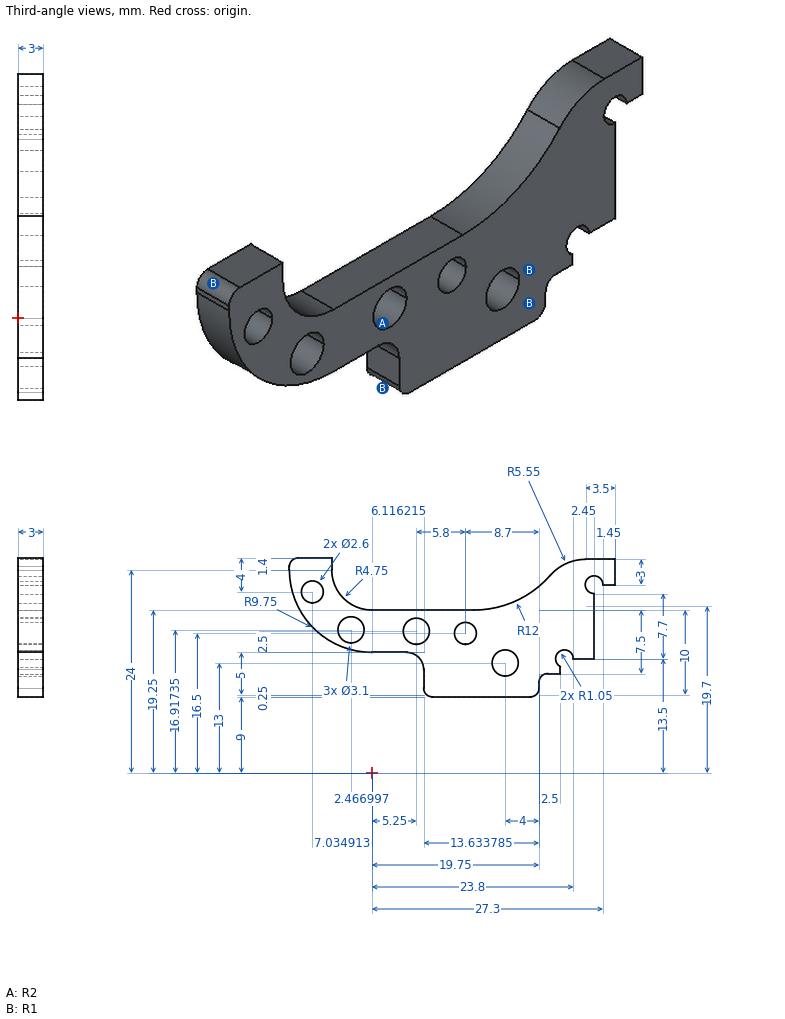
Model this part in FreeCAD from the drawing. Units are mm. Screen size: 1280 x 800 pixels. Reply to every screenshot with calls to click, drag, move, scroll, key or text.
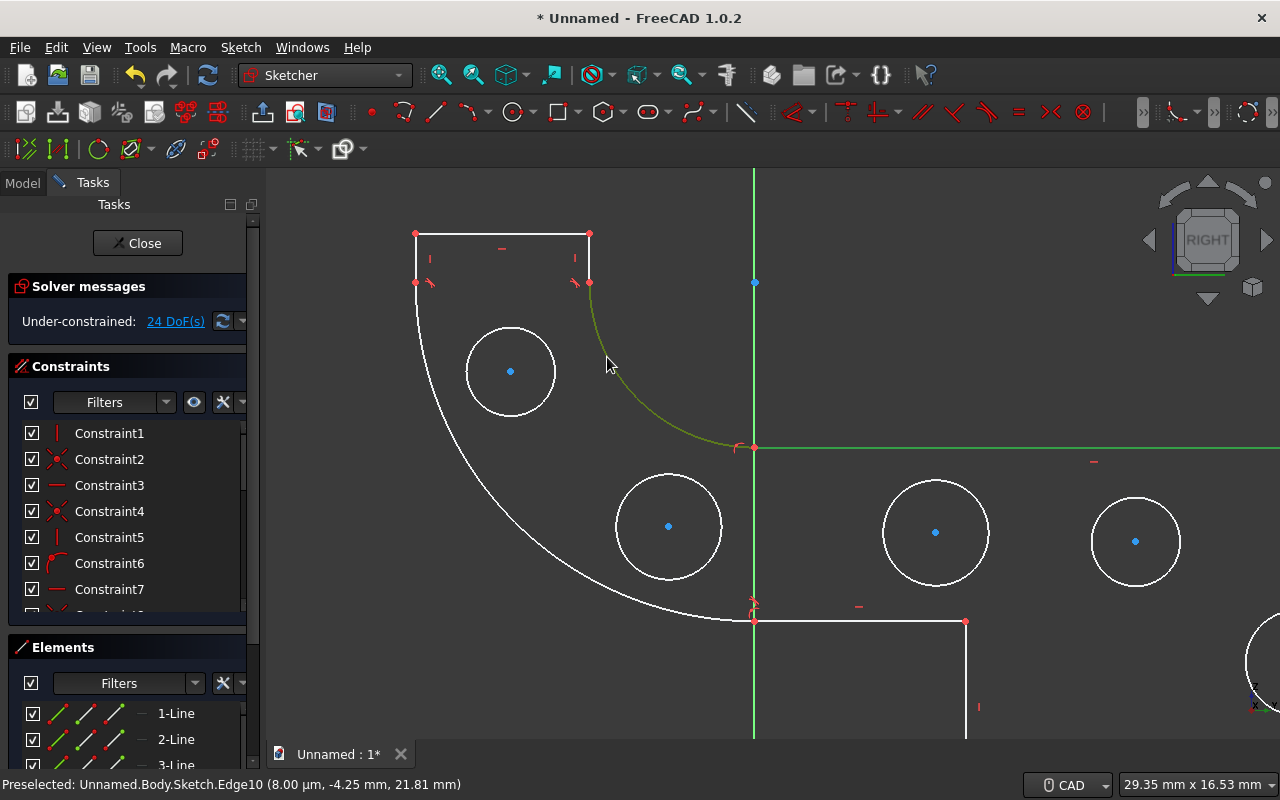
key(t)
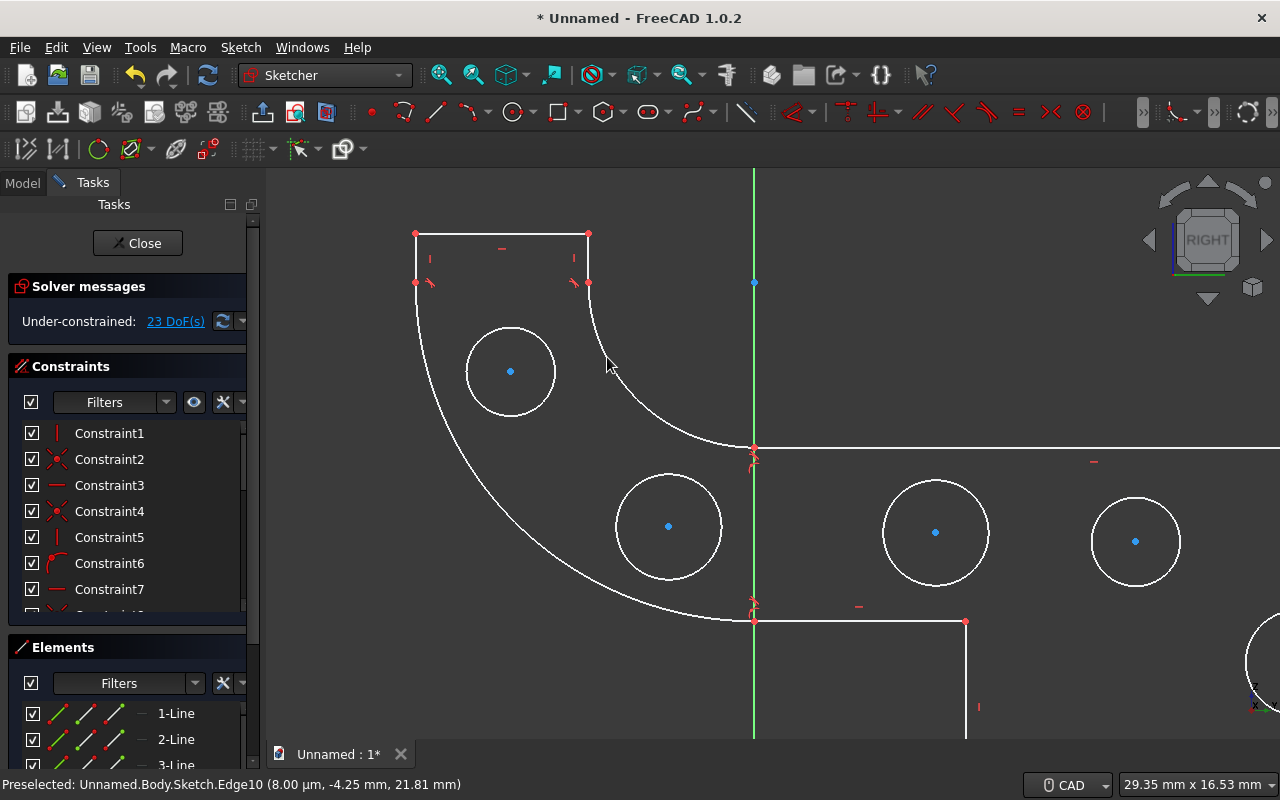
click(706, 490)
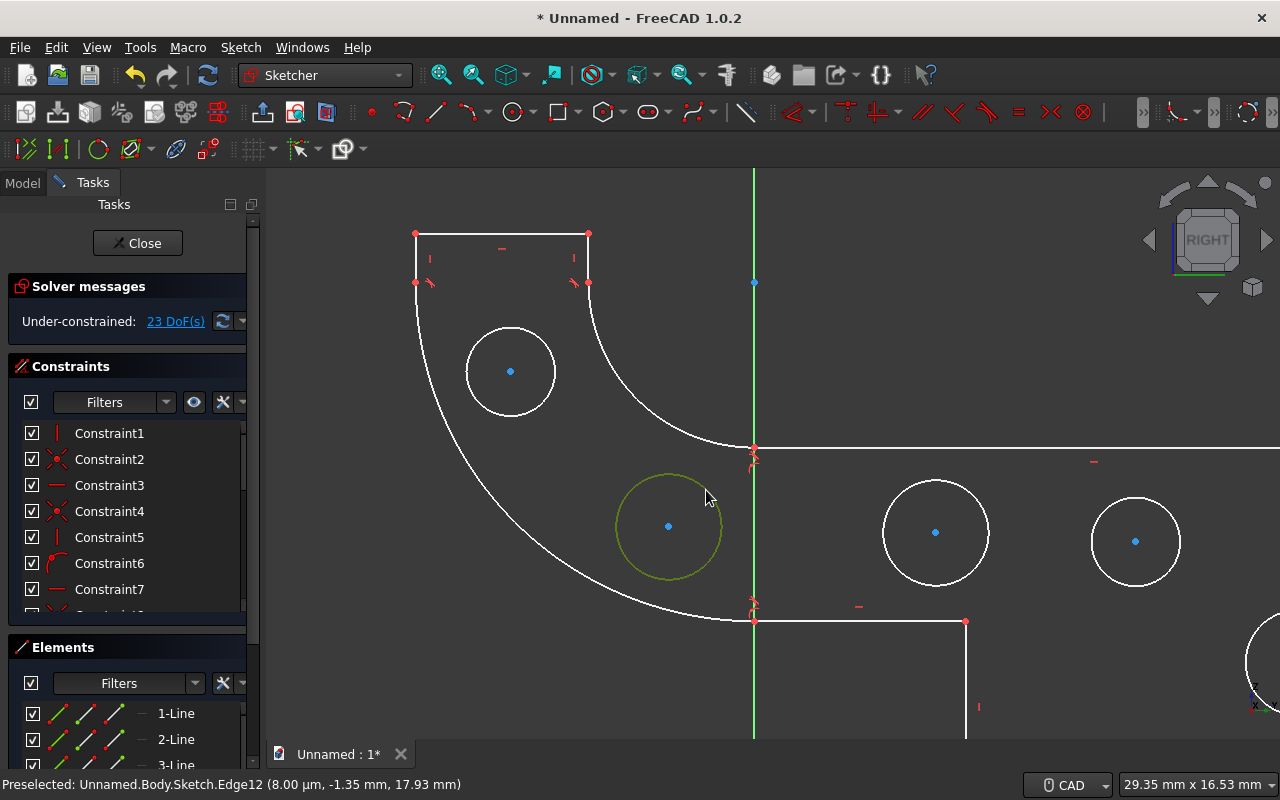
click(973, 496)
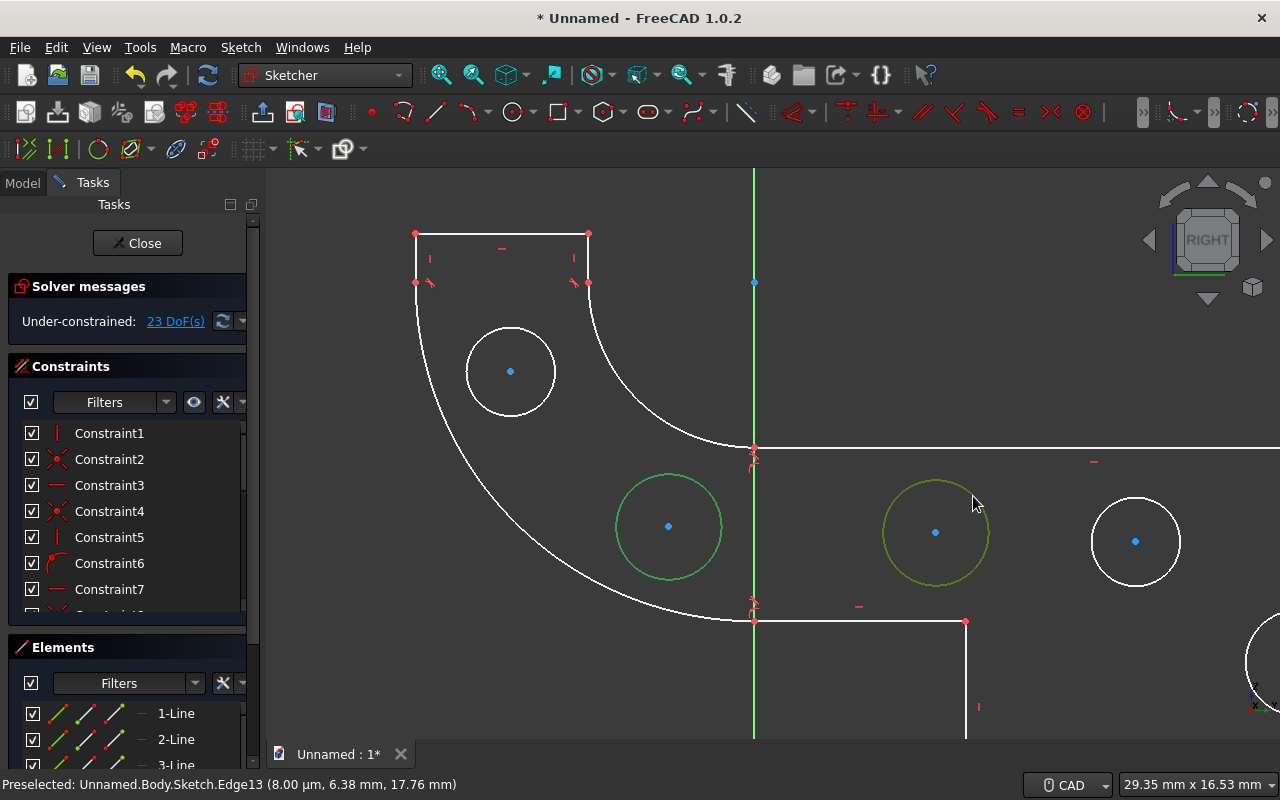
scroll(523, 276, down, 4)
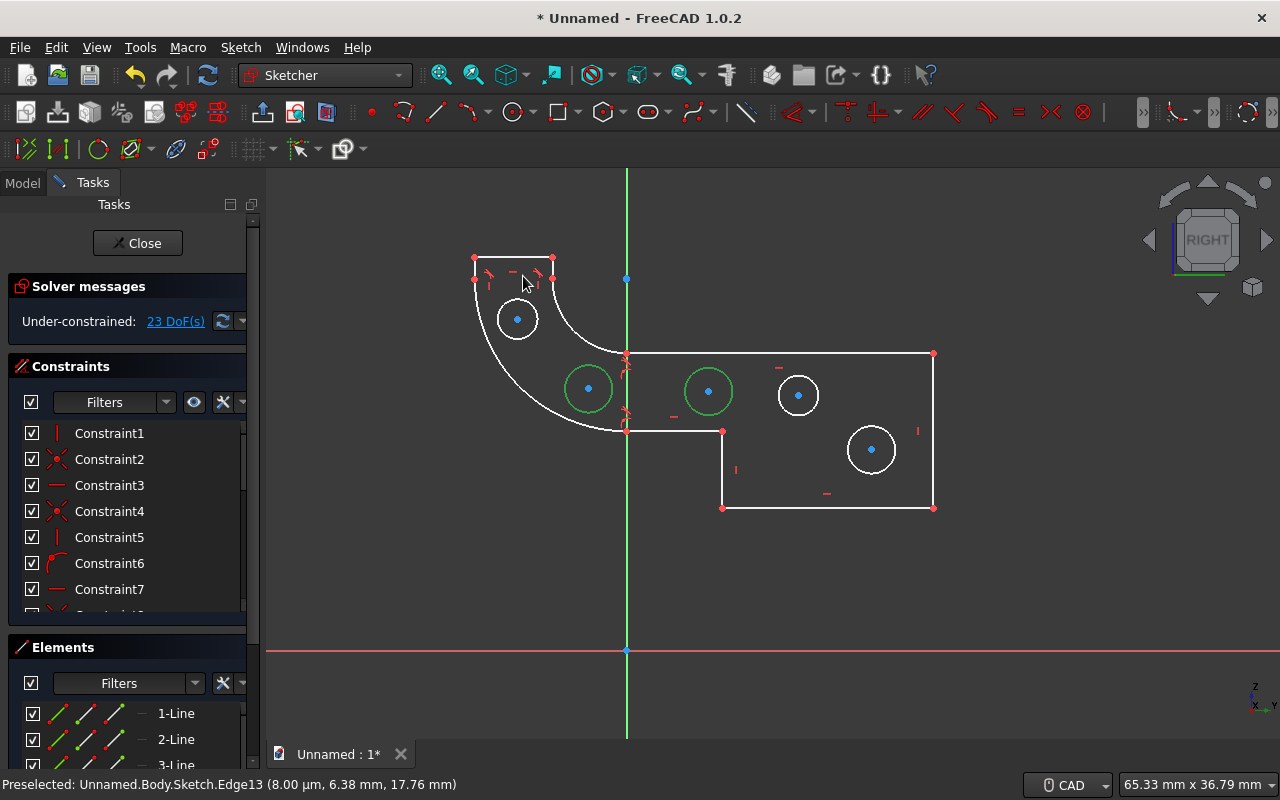
click(888, 433)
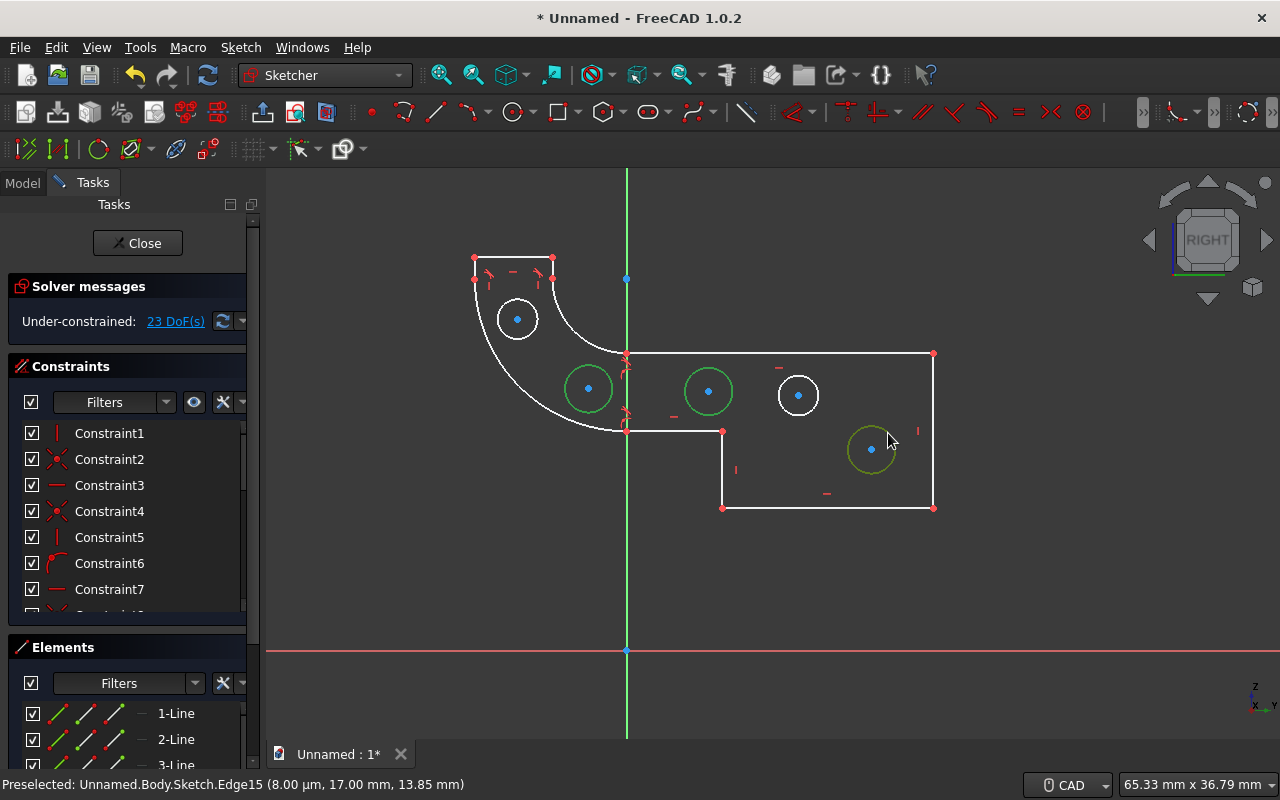
key(e)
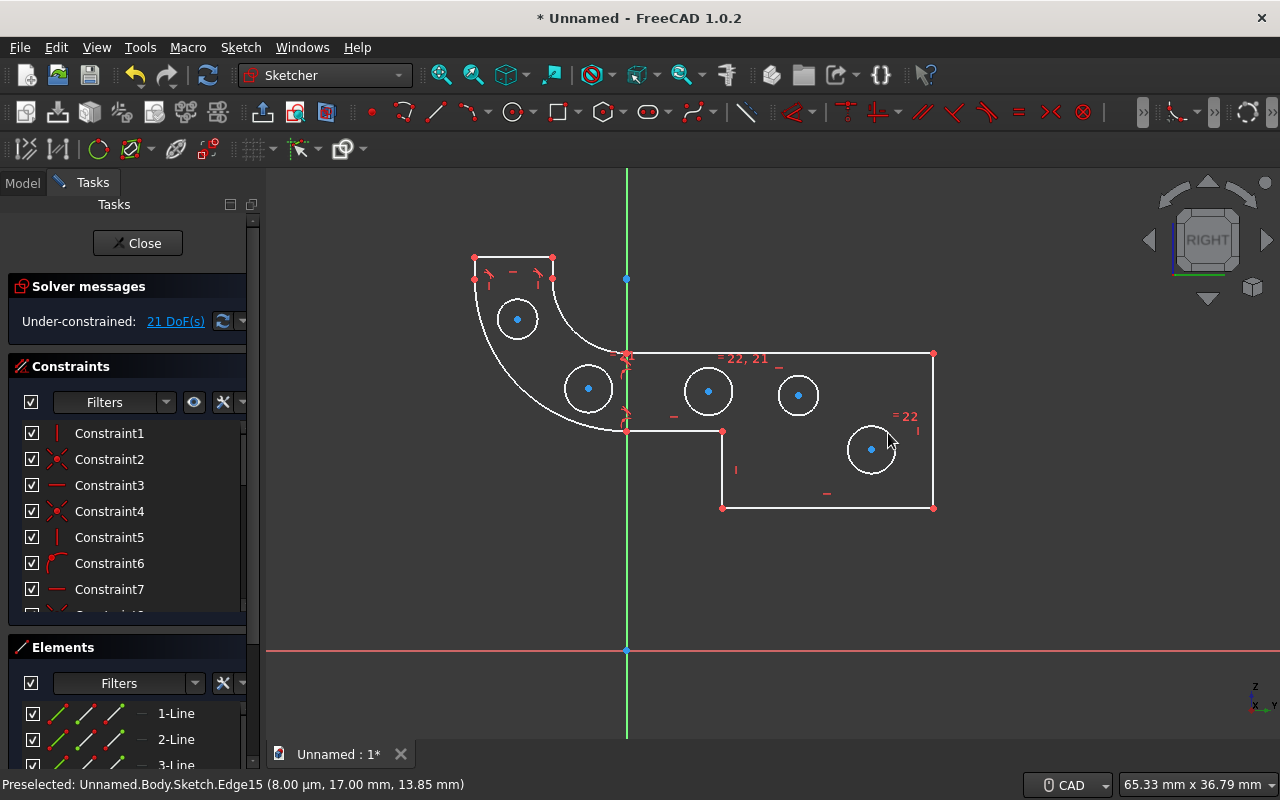
click(532, 305)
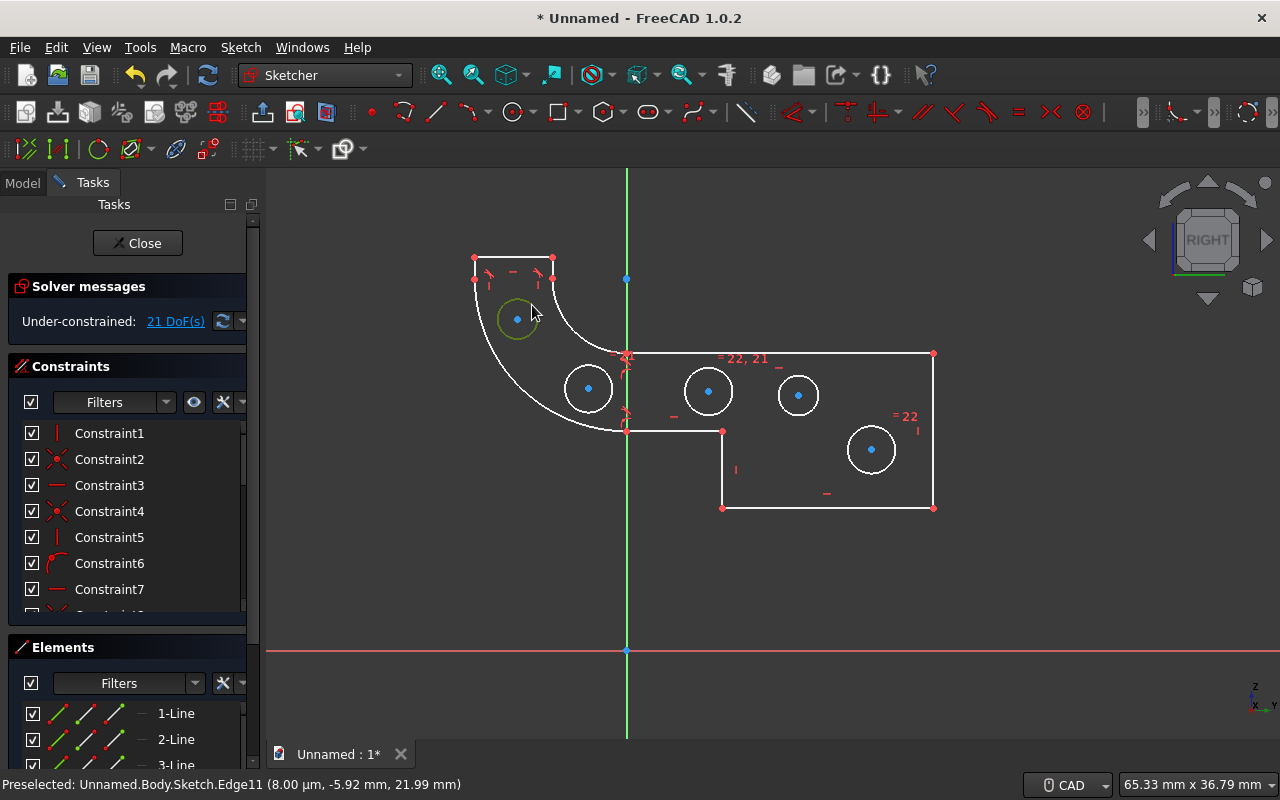
click(813, 381)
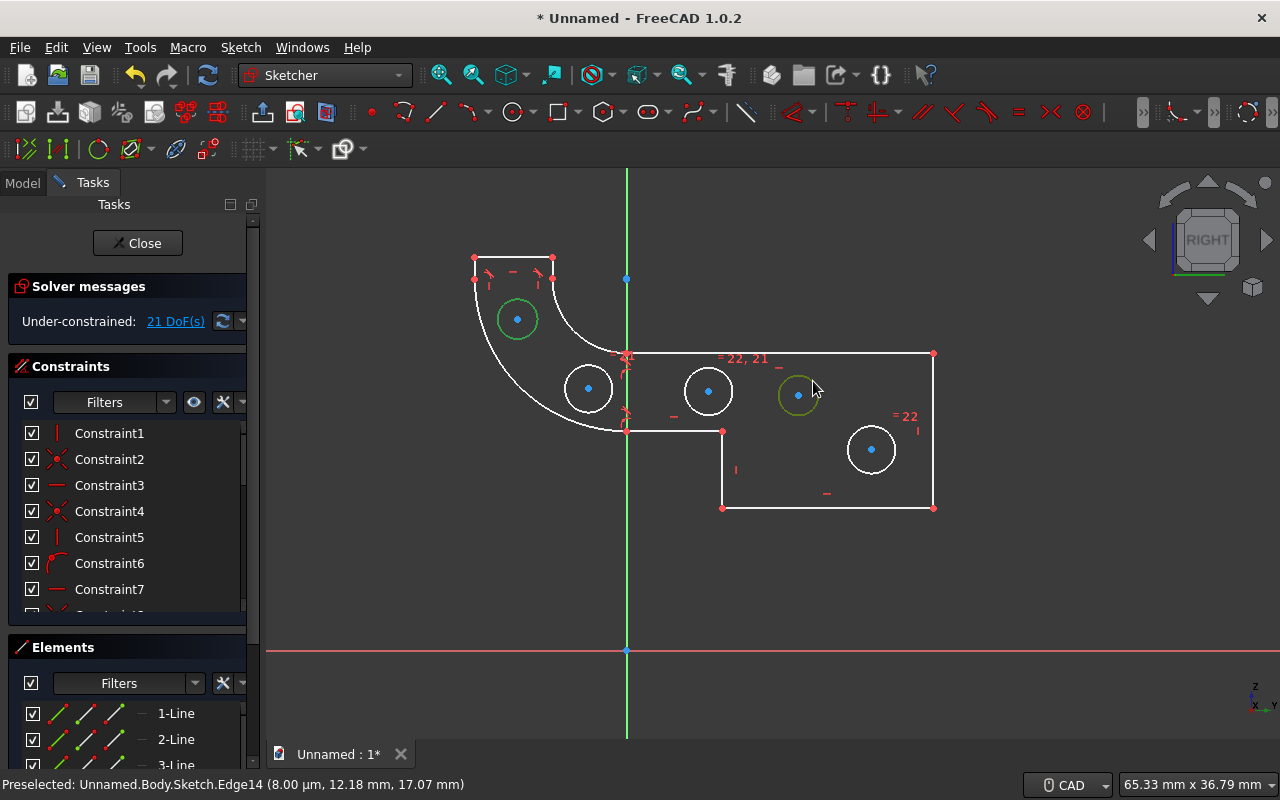
key(e)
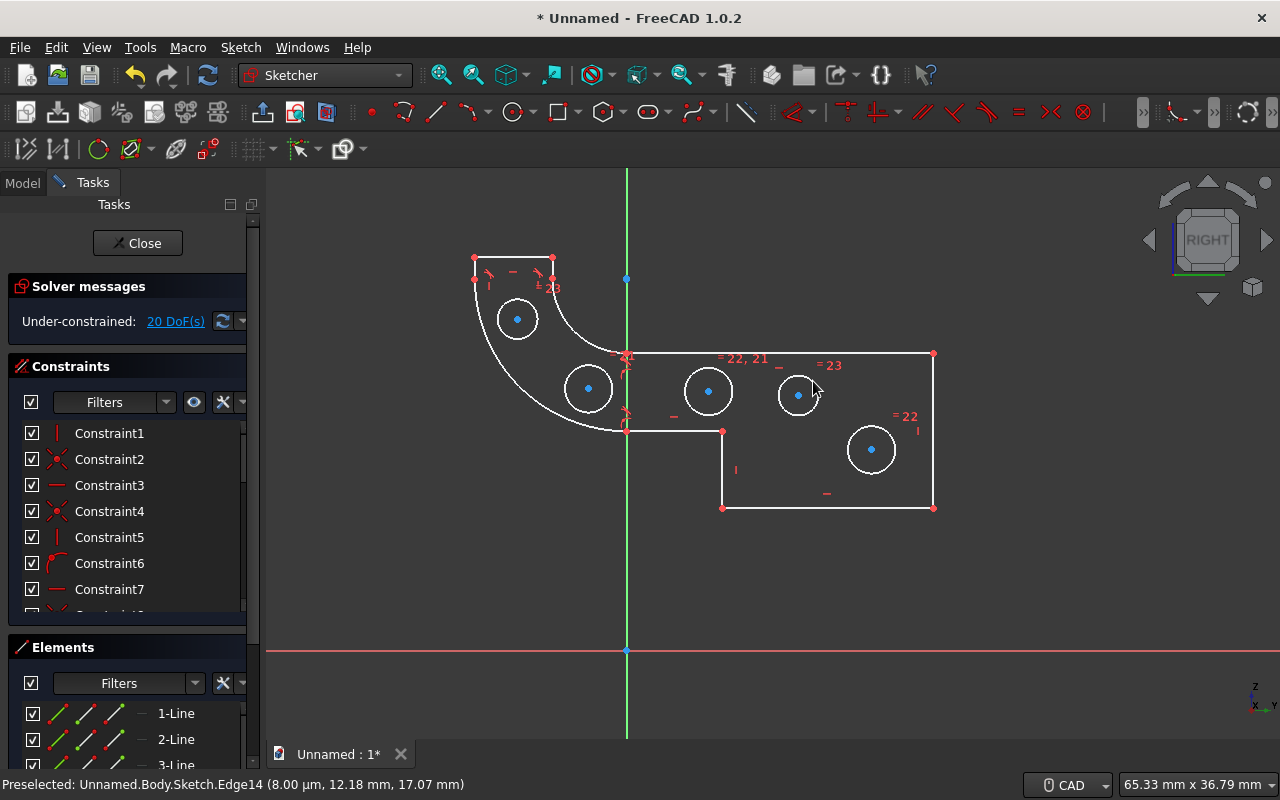
click(792, 112)